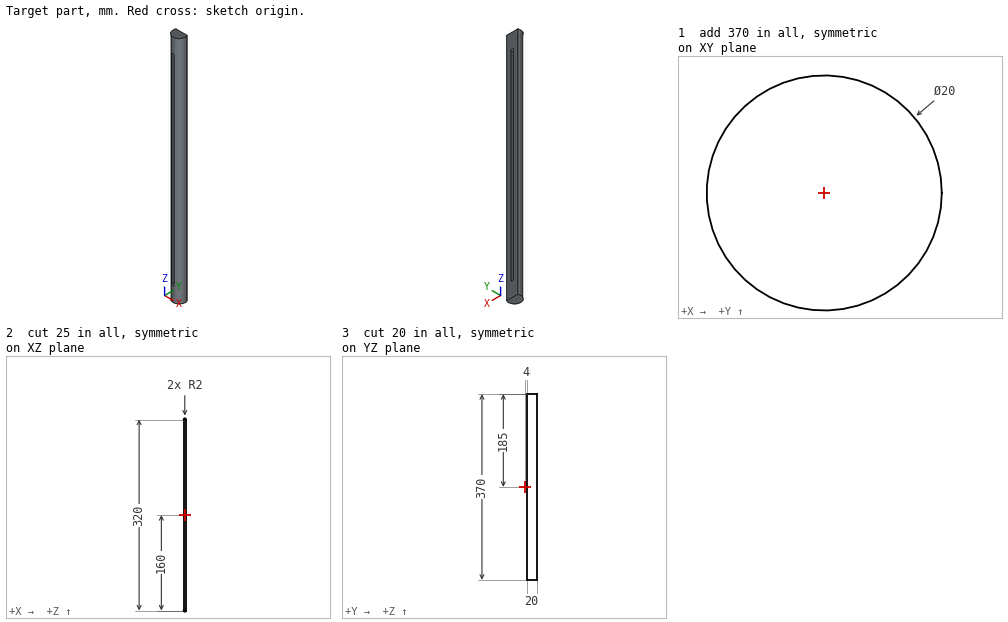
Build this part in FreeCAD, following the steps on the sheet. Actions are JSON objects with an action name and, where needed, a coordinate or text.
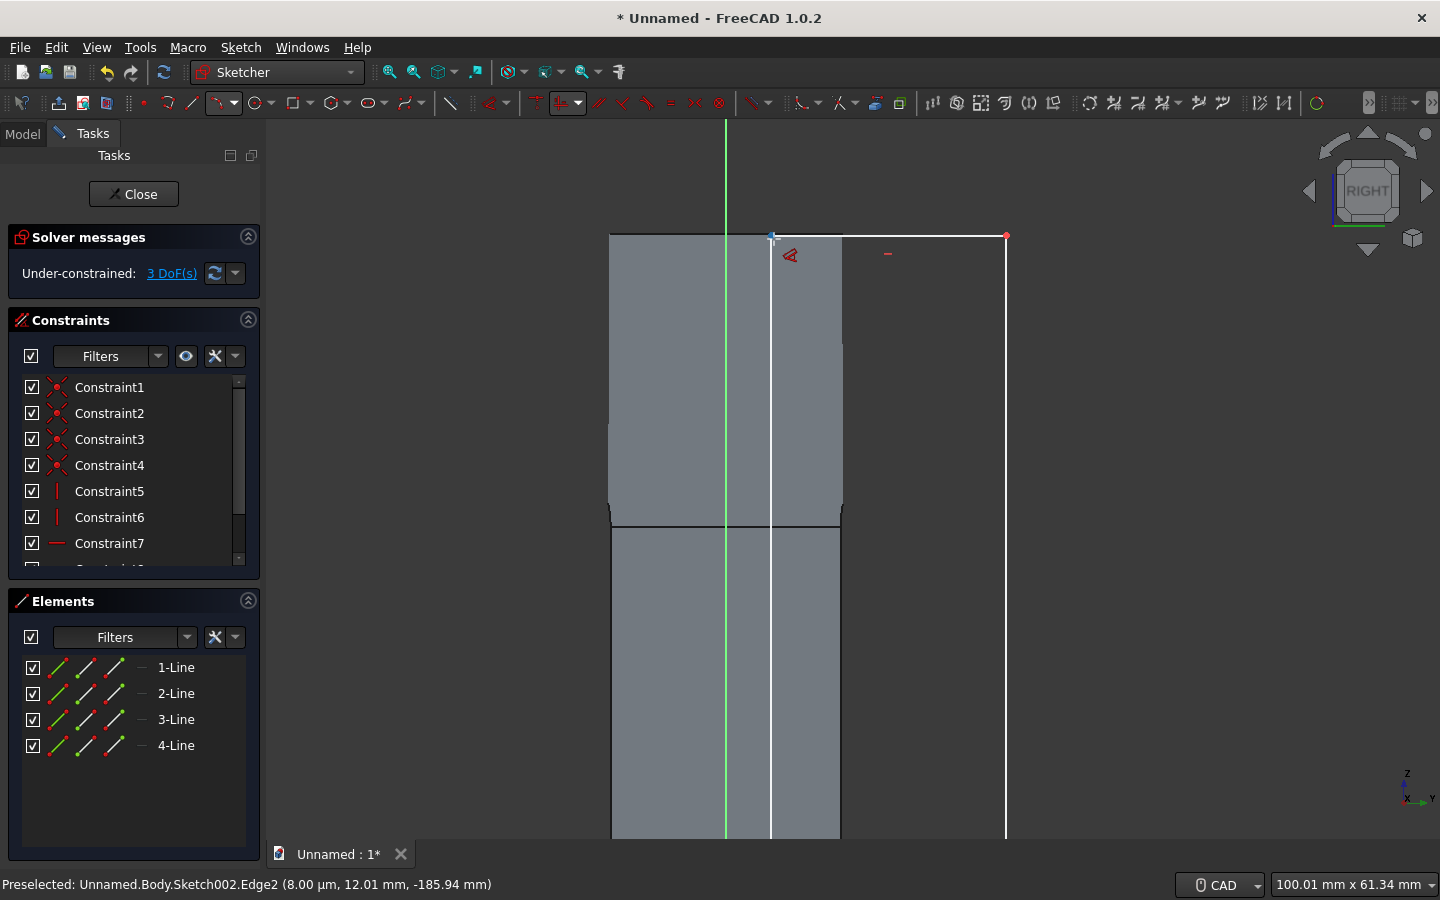
{"action": "left_click", "coordinate": [771, 236]}
{"action": "left_click", "coordinate": [748, 202]}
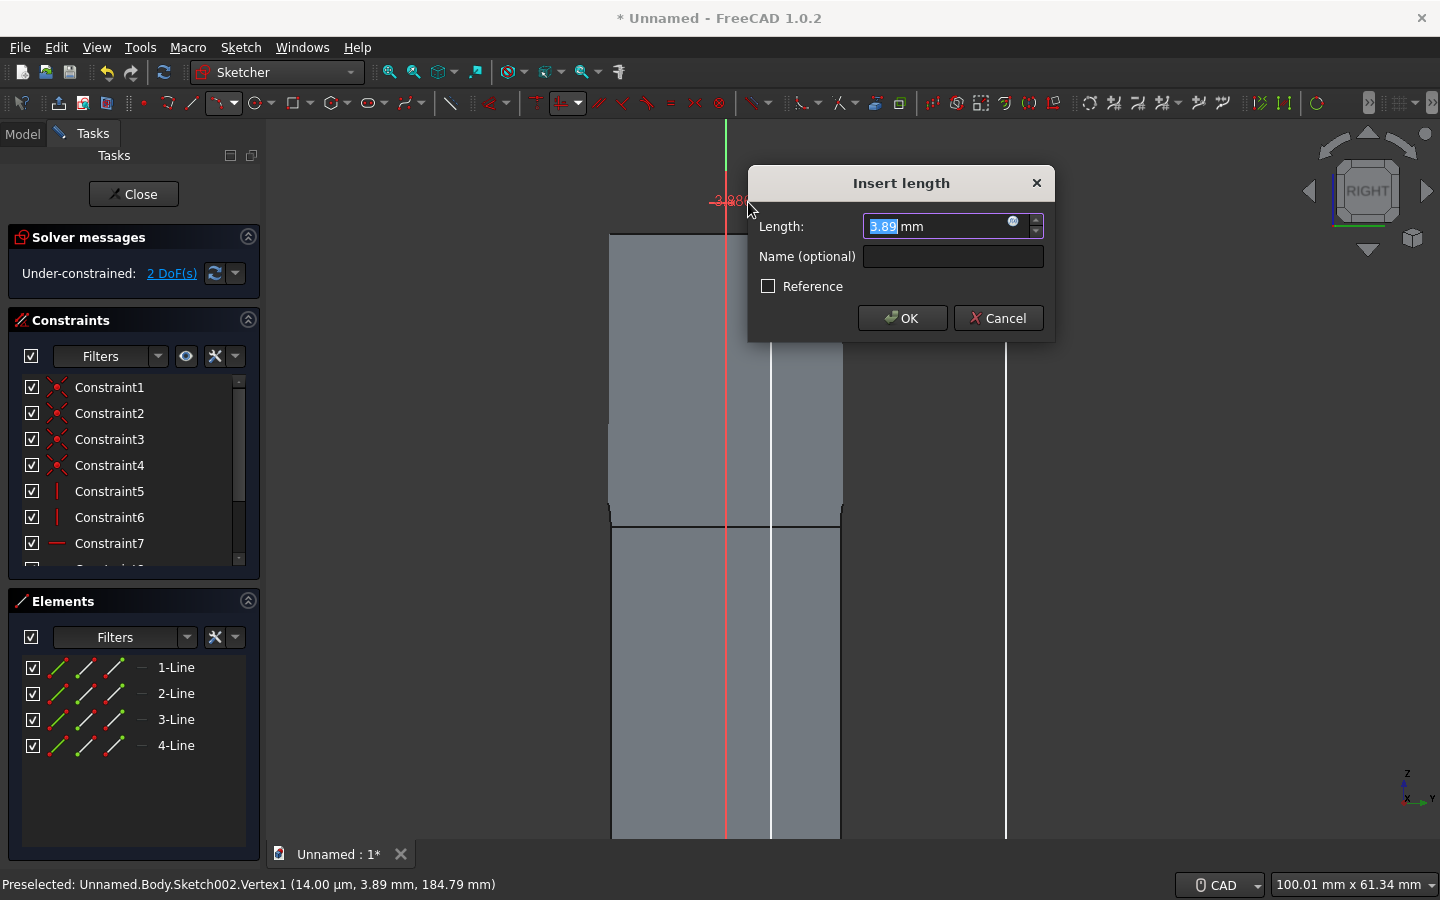
{"action": "type", "text": "4"}
{"action": "key", "text": "Return"}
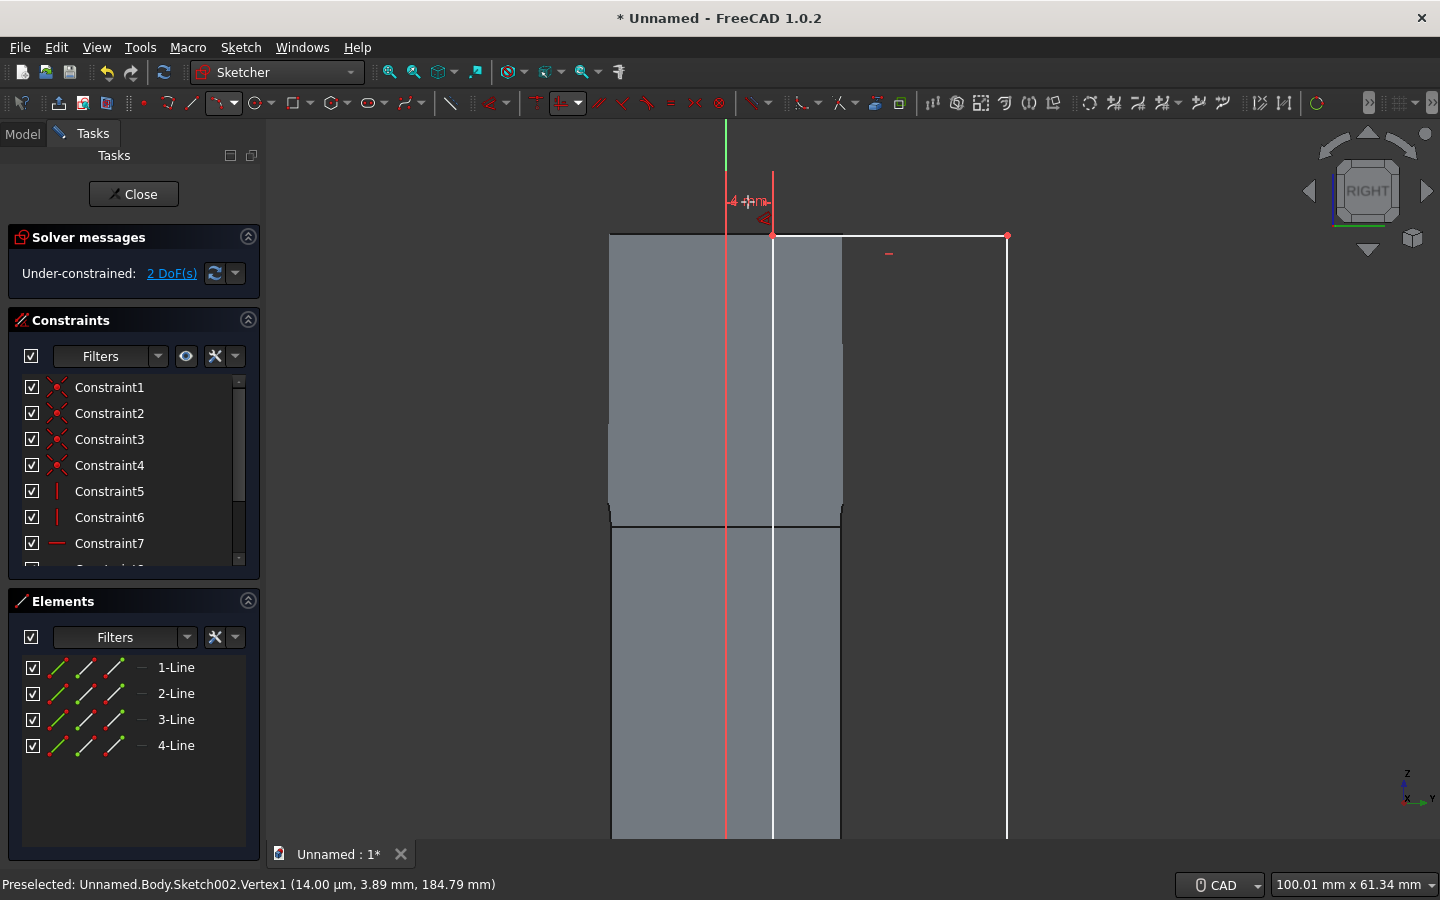
{"action": "scroll", "coordinate": [774, 239], "scroll_direction": "down", "scroll_amount": 11}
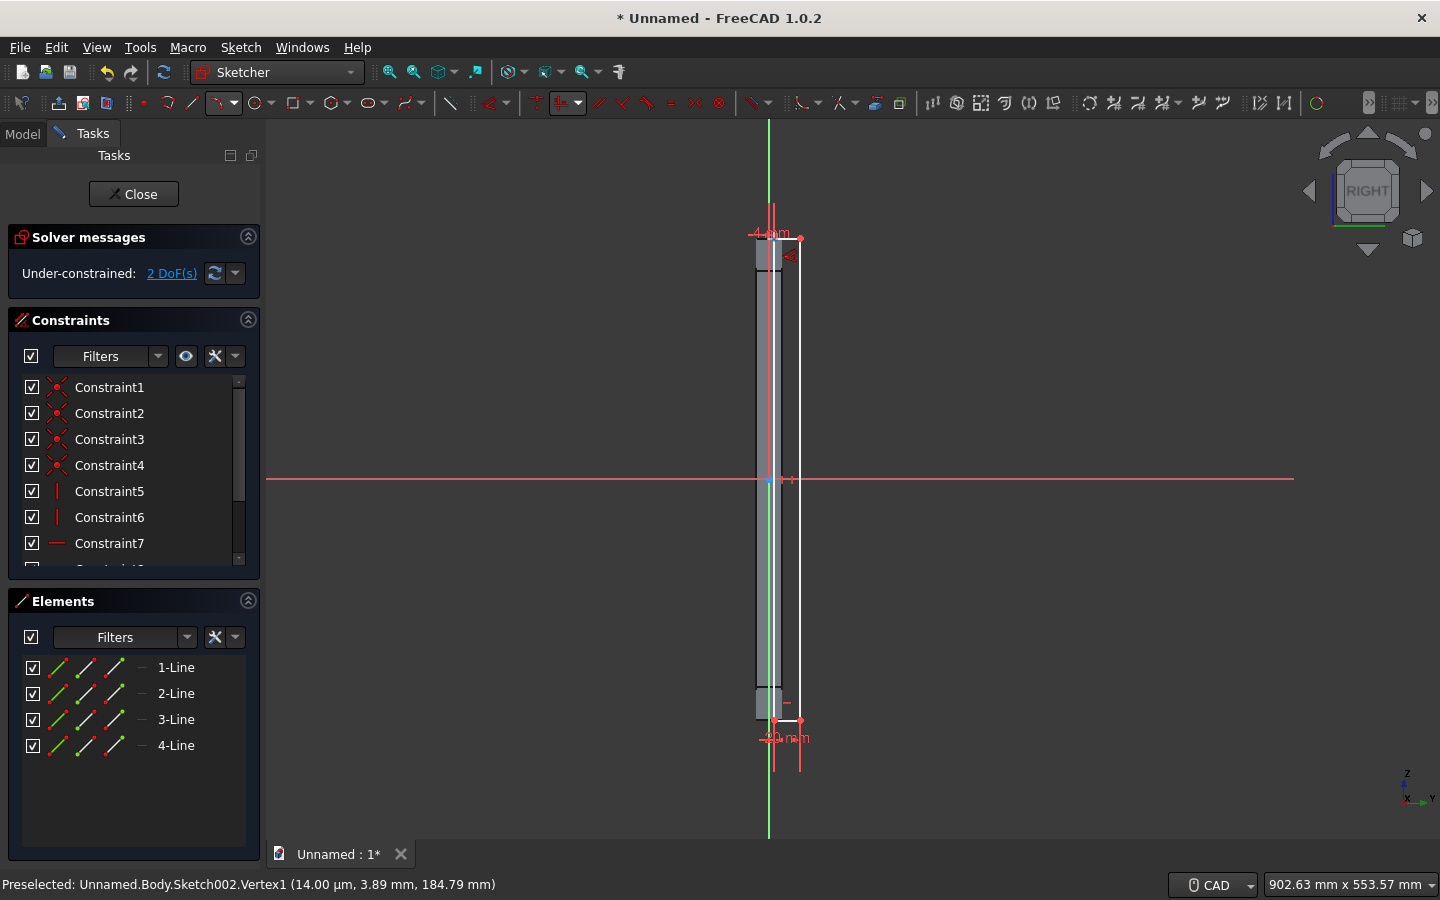
{"action": "scroll", "coordinate": [774, 383], "scroll_direction": "up", "scroll_amount": 5}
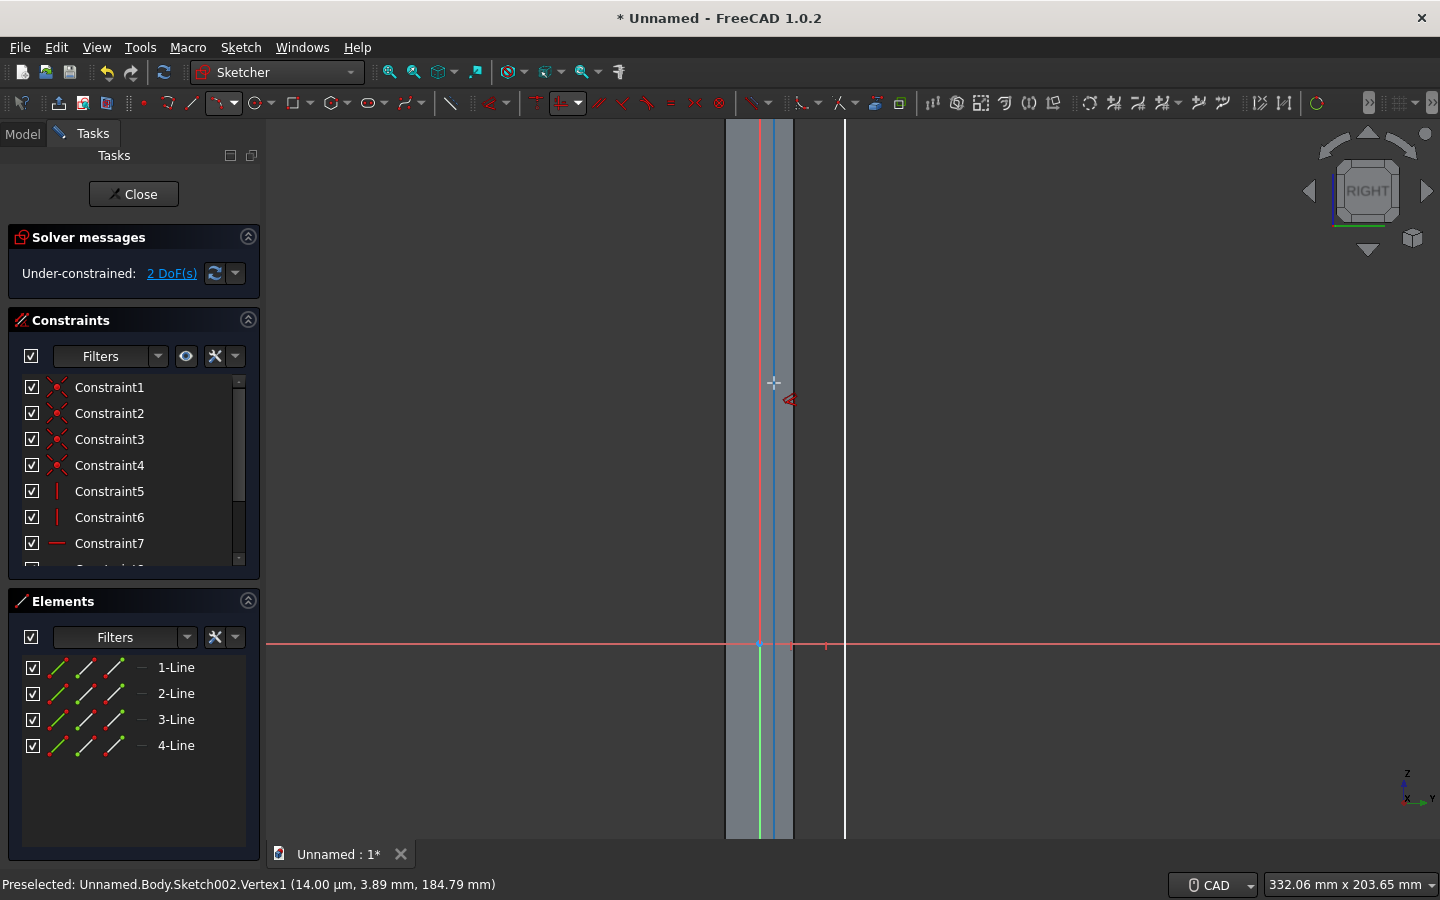
{"action": "left_click", "coordinate": [774, 384]}
{"action": "left_click", "coordinate": [740, 479]}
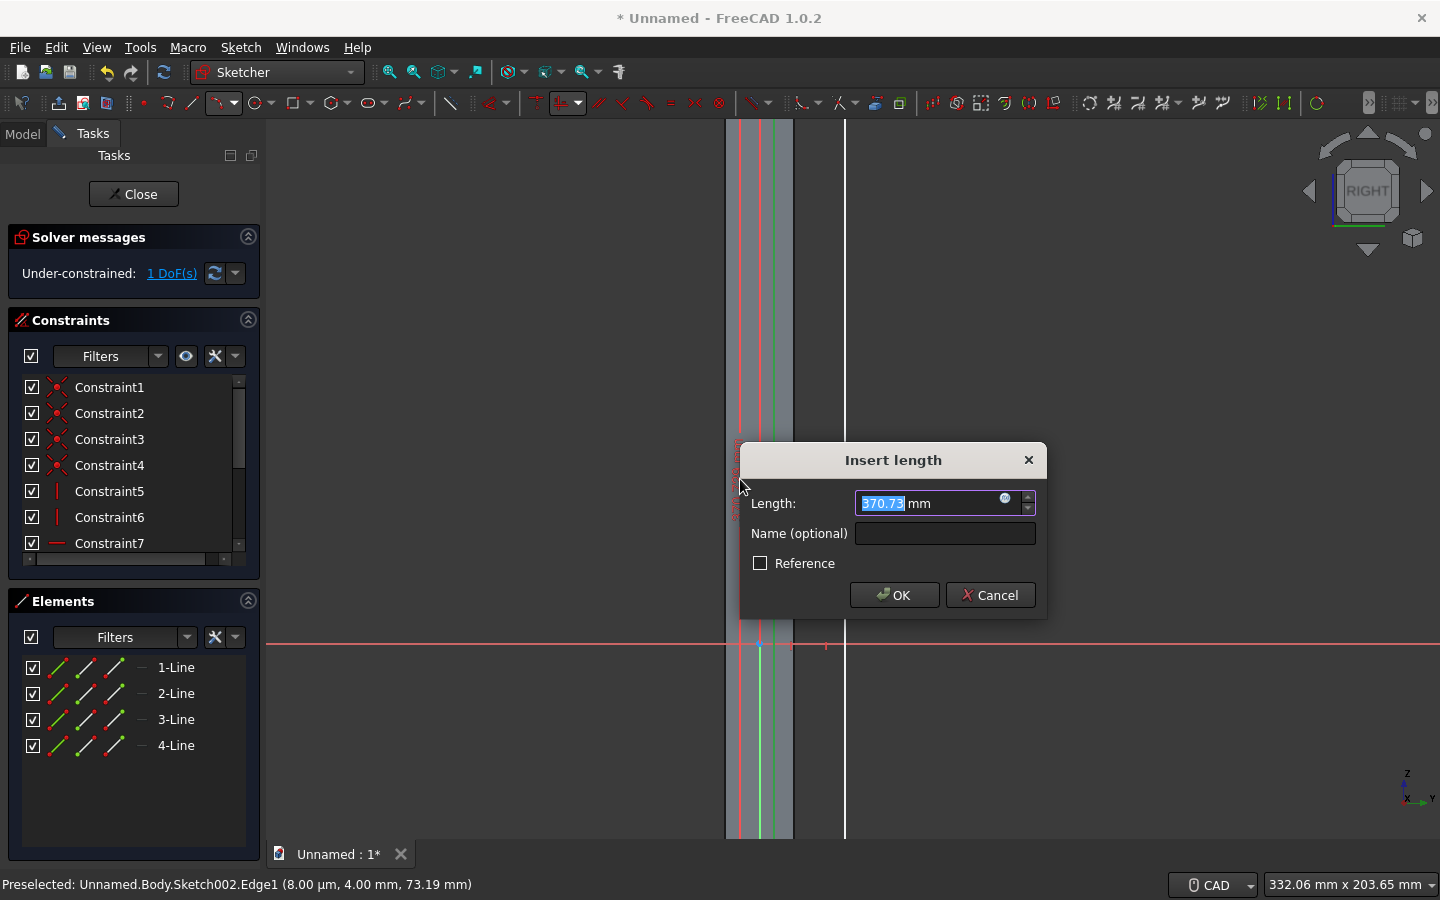
{"action": "type", "text": "370"}
{"action": "key", "text": "Return"}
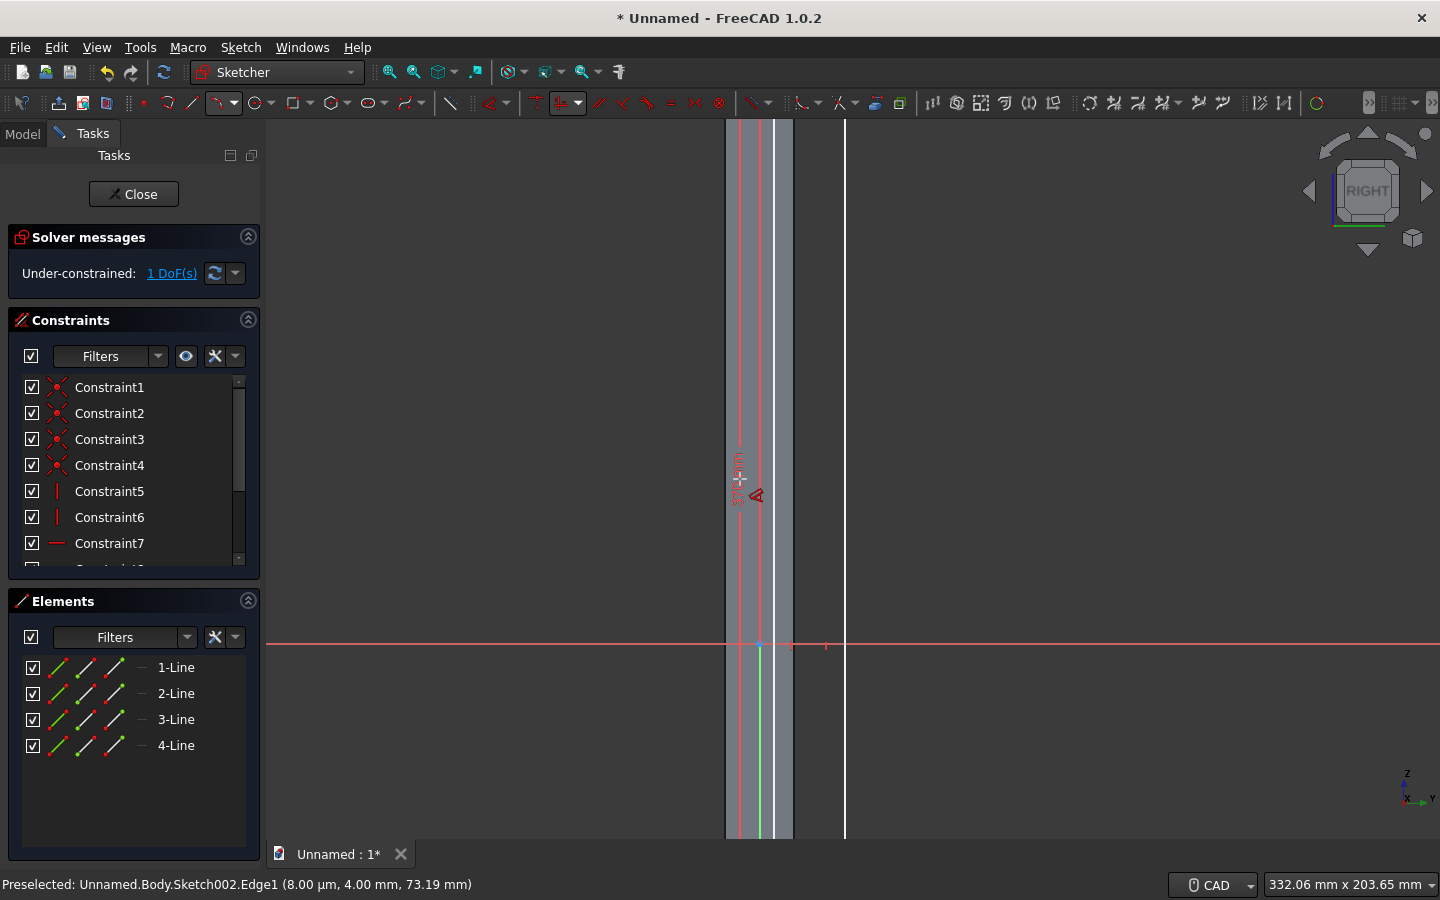
{"action": "scroll", "coordinate": [774, 383], "scroll_direction": "down", "scroll_amount": 5}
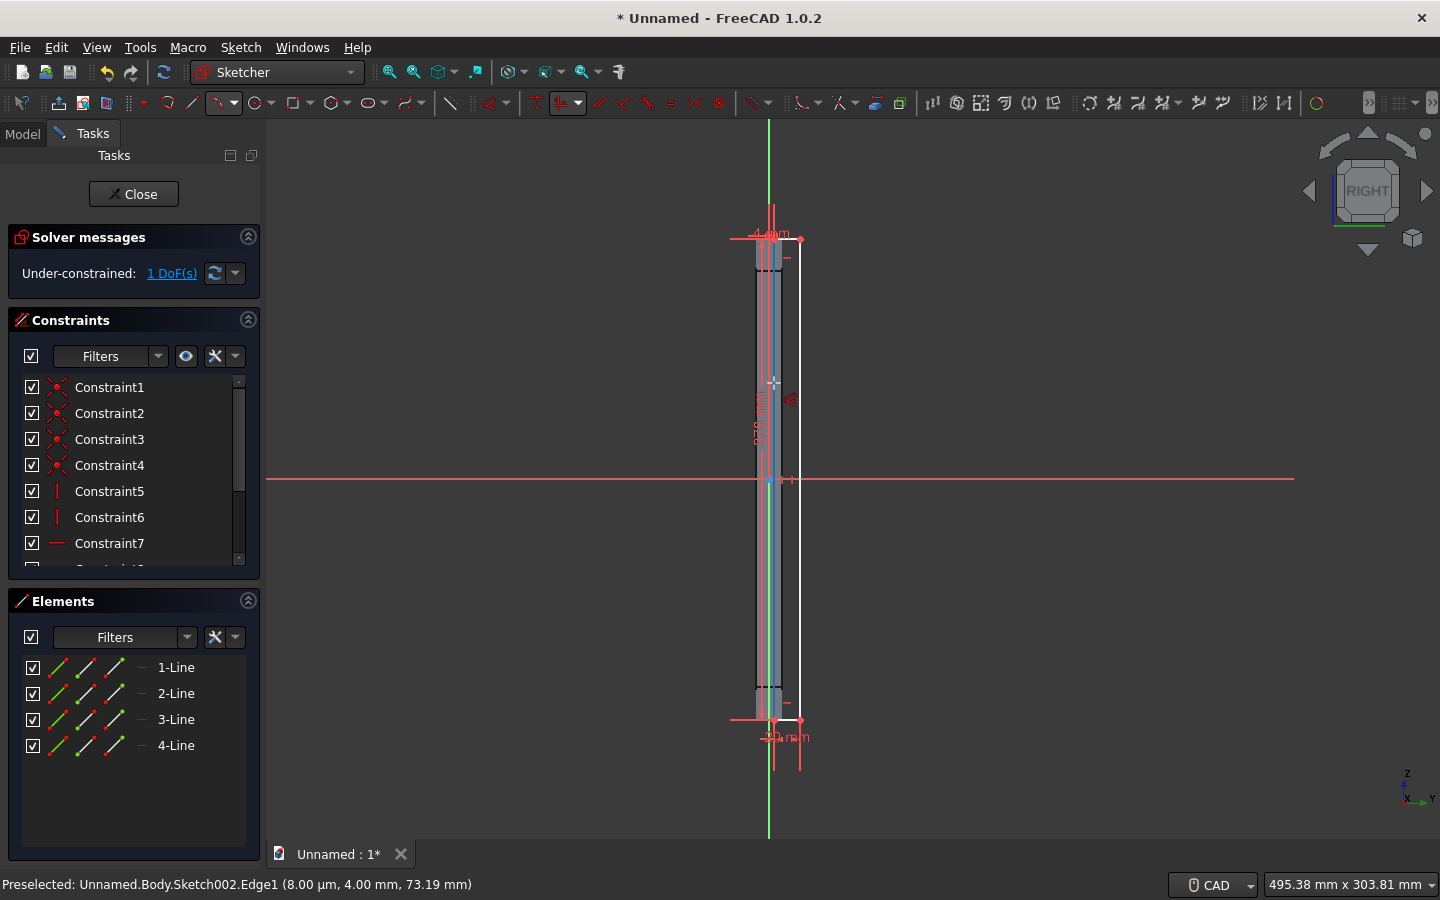
{"action": "left_click", "coordinate": [774, 239]}
{"action": "left_click", "coordinate": [735, 359]}